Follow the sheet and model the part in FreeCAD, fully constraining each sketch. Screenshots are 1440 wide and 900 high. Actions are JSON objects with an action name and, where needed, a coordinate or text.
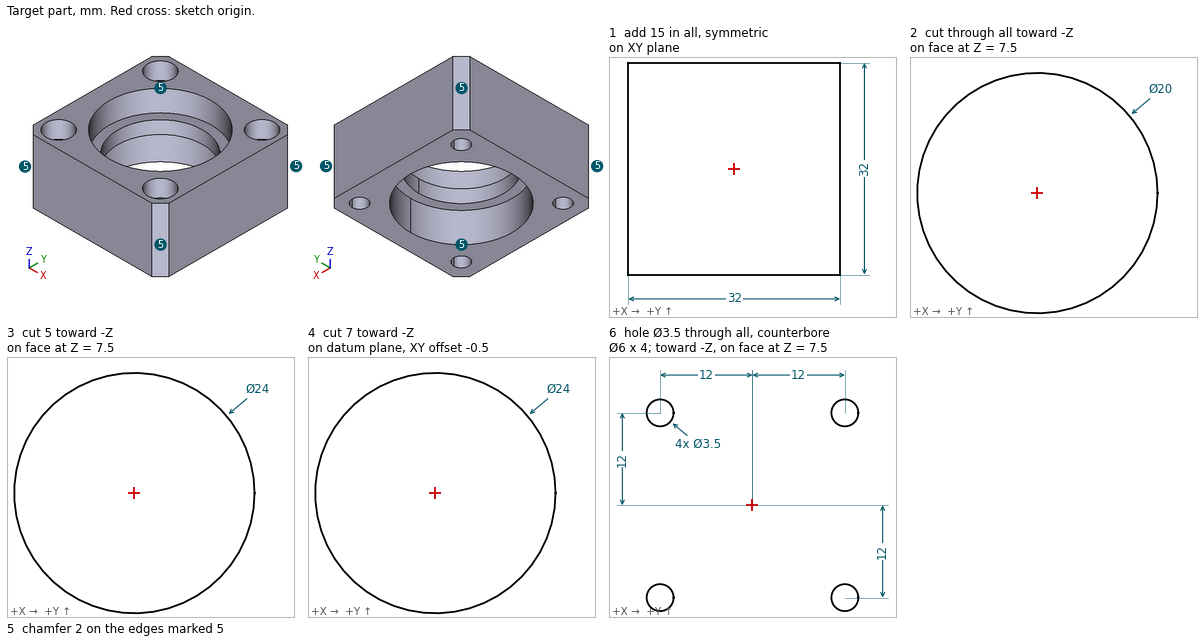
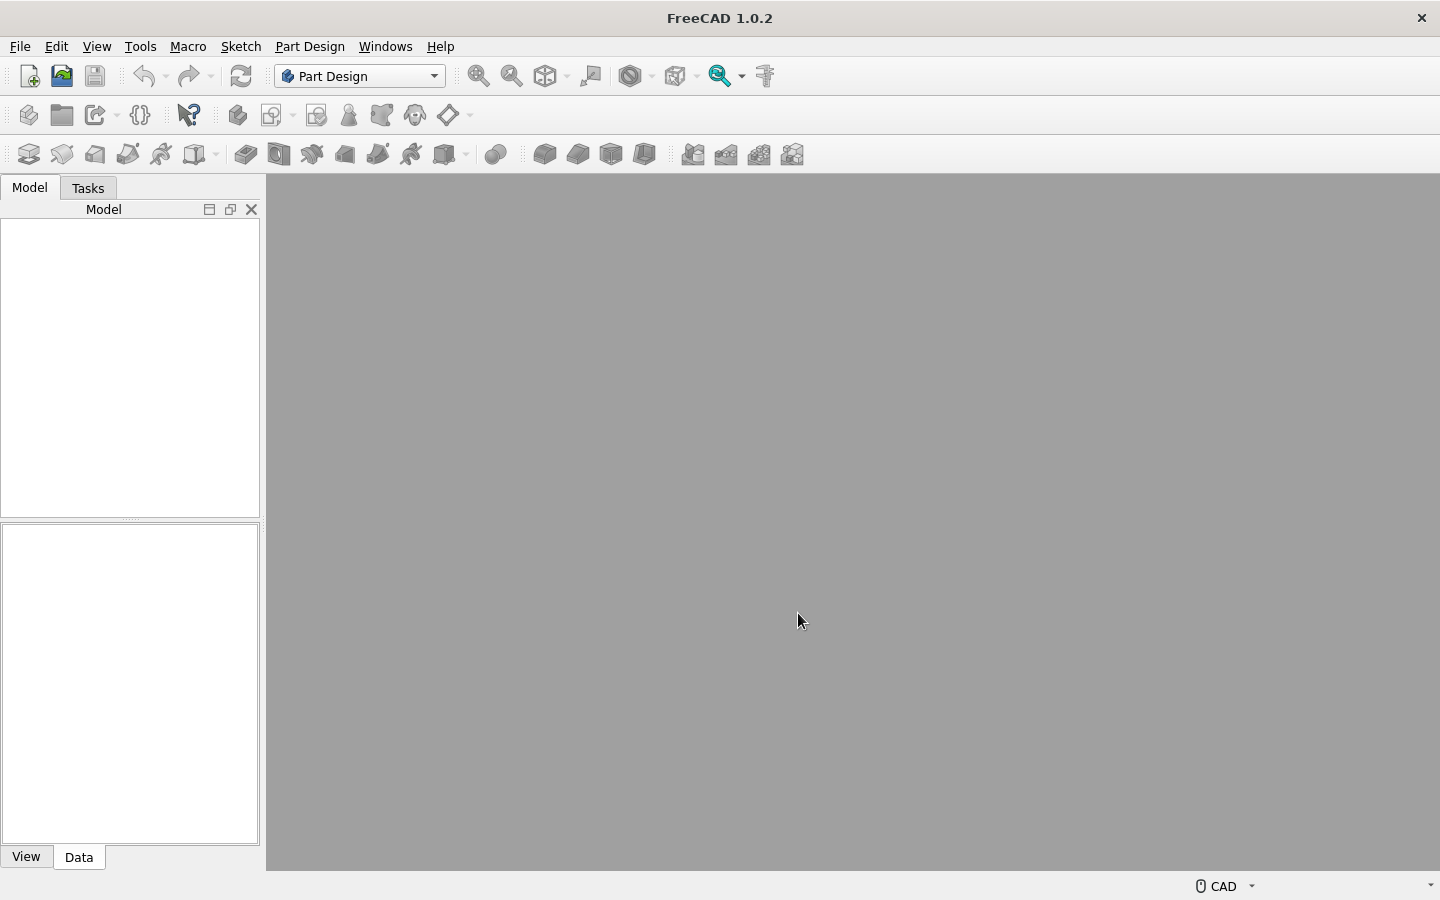
{"action": "left_click", "coordinate": [29, 76]}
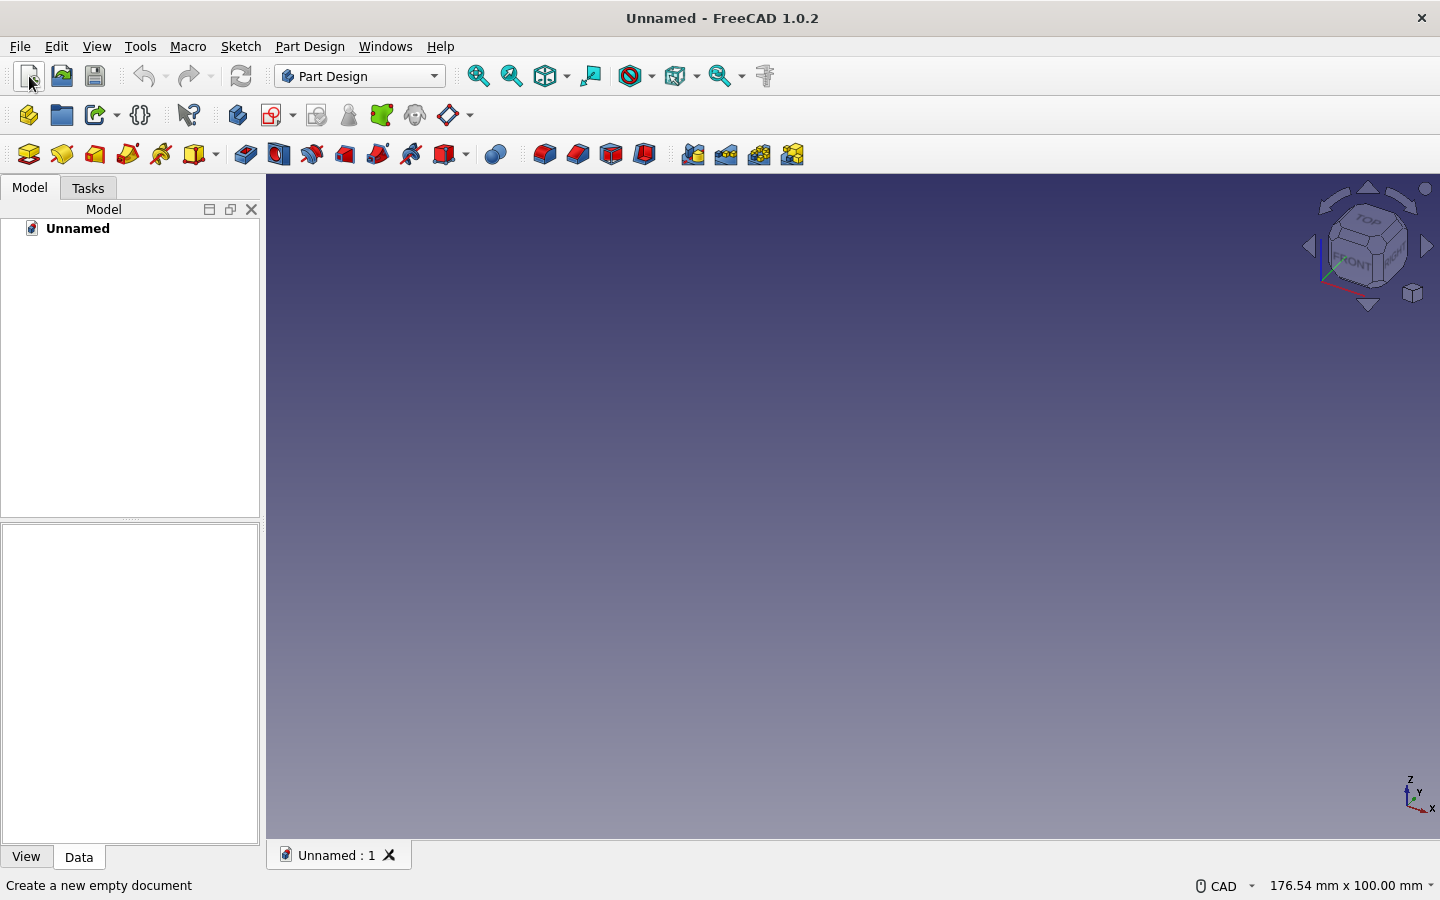
{"action": "left_click", "coordinate": [270, 116]}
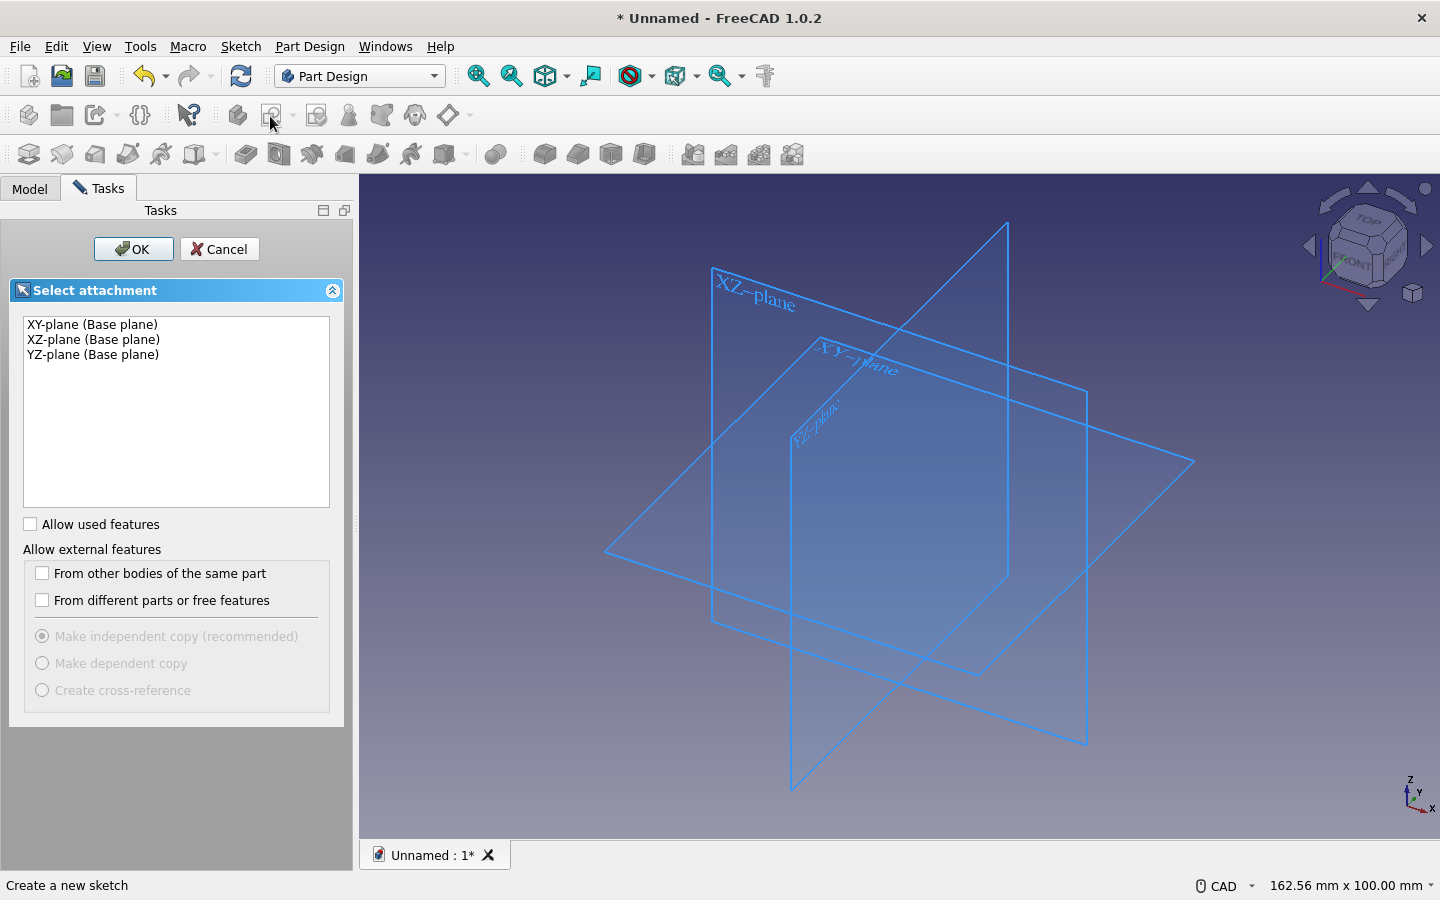
{"action": "left_click", "coordinate": [84, 324]}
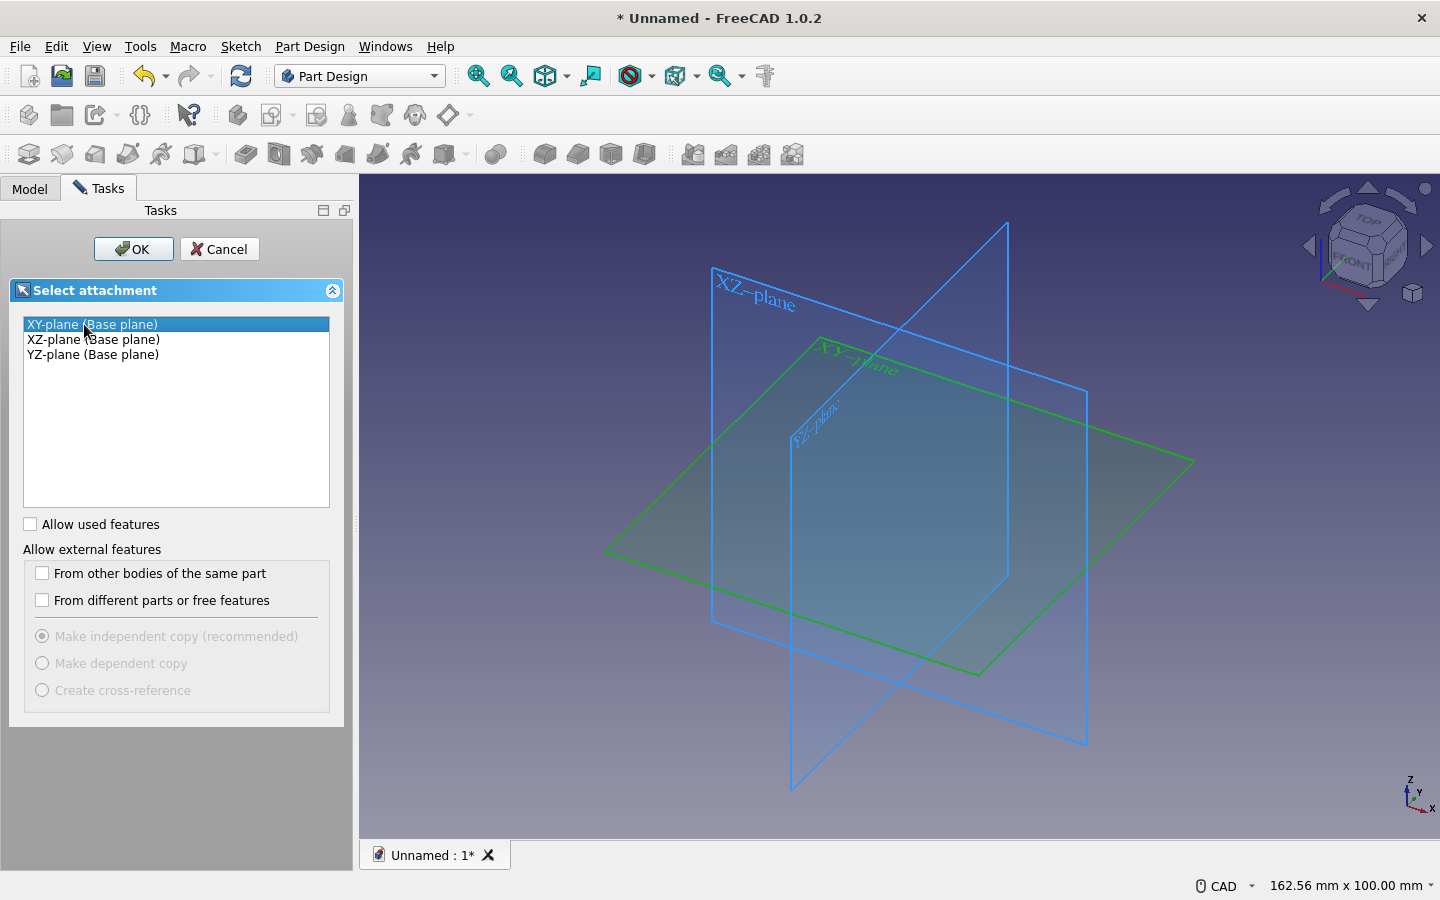
{"action": "left_click", "coordinate": [134, 249]}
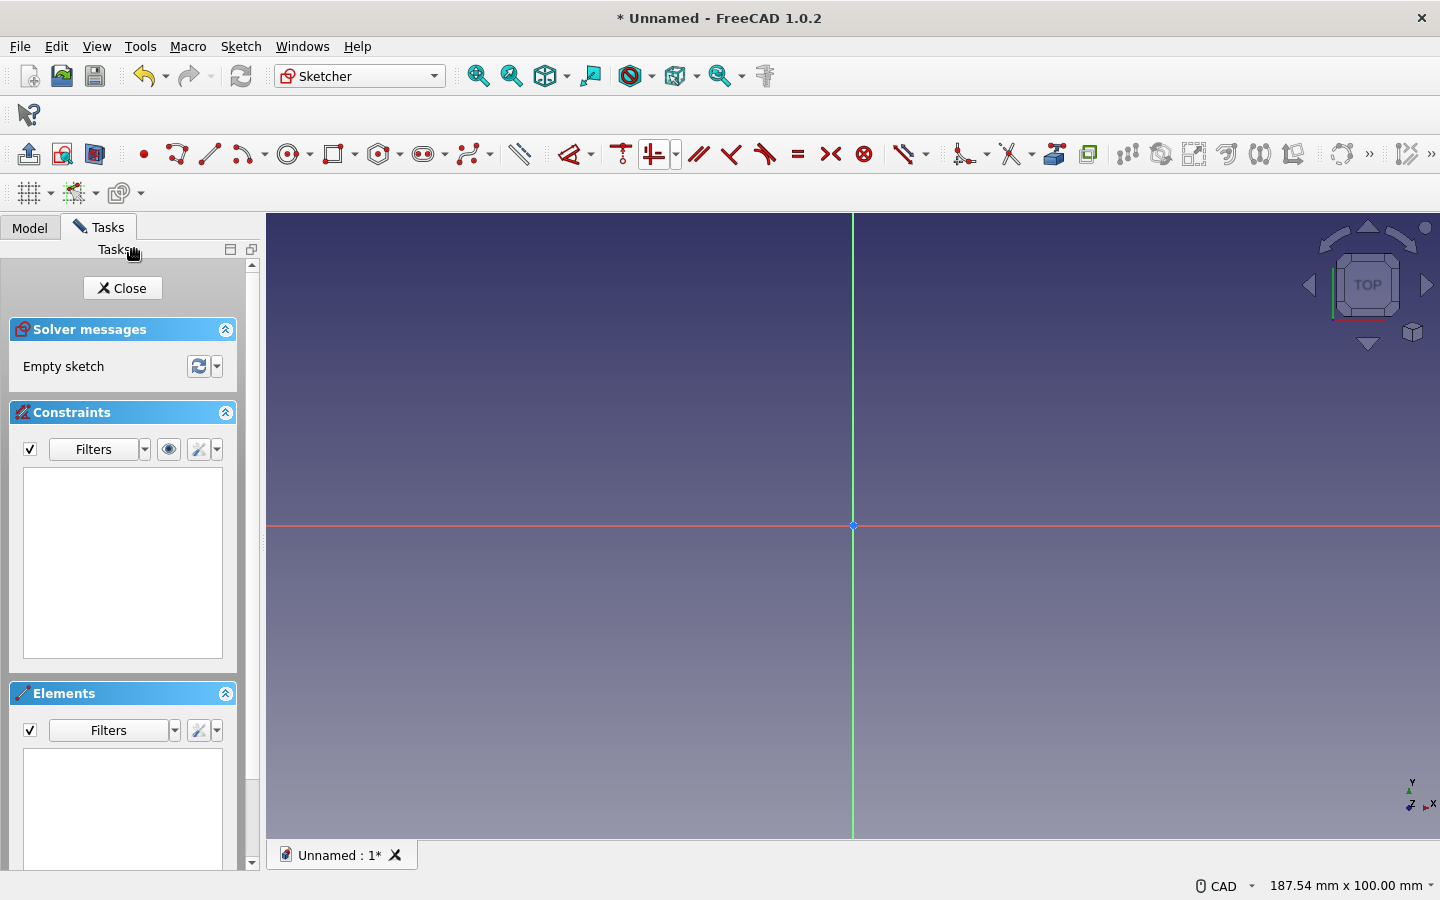
{"action": "scroll", "coordinate": [936, 526], "scroll_direction": "up", "scroll_amount": 3}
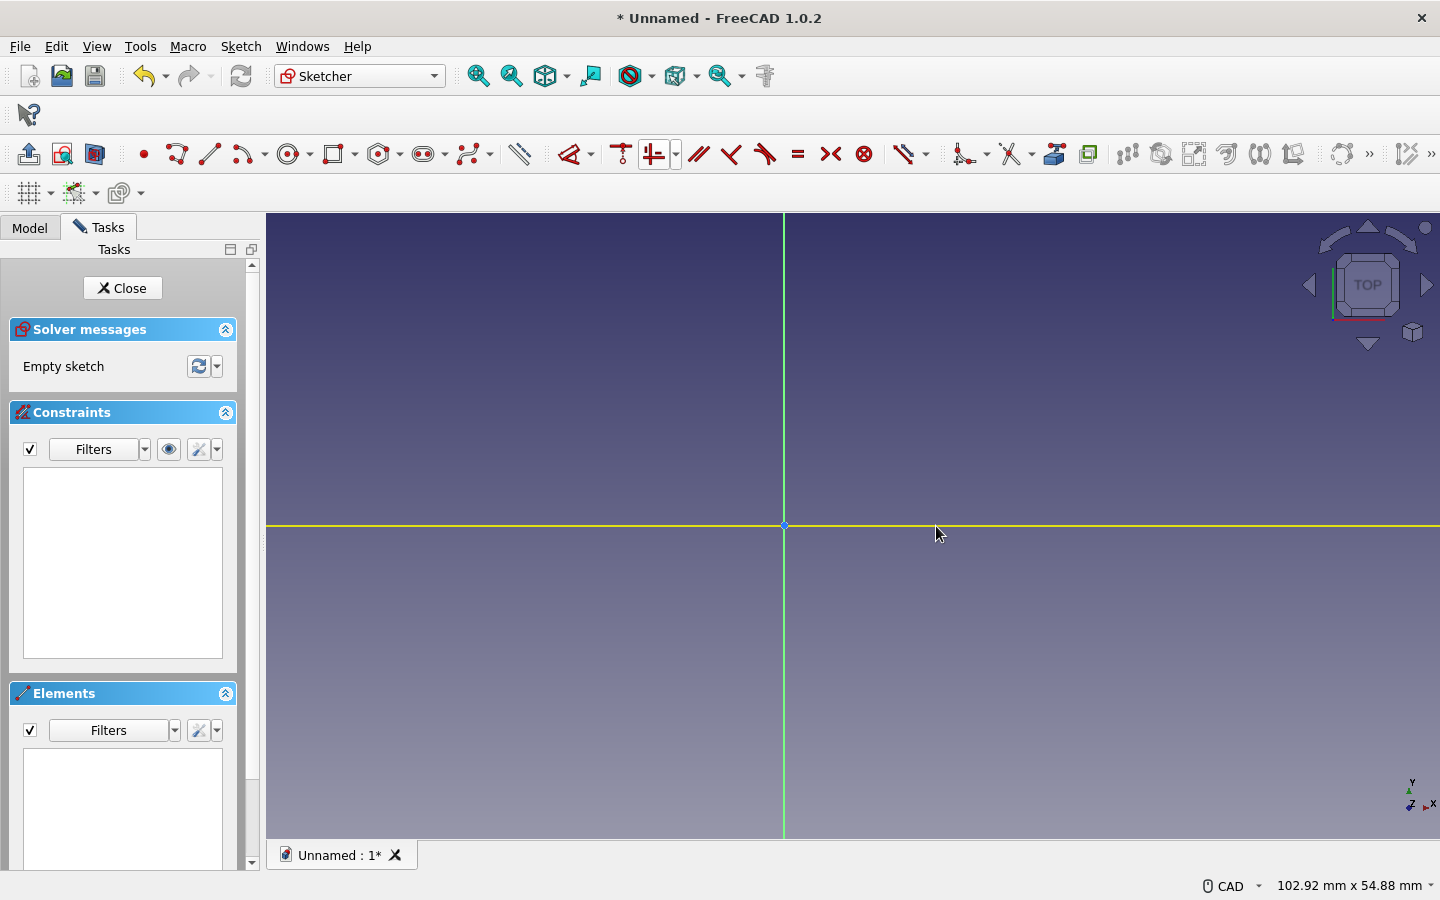
{"action": "key", "text": "g v"}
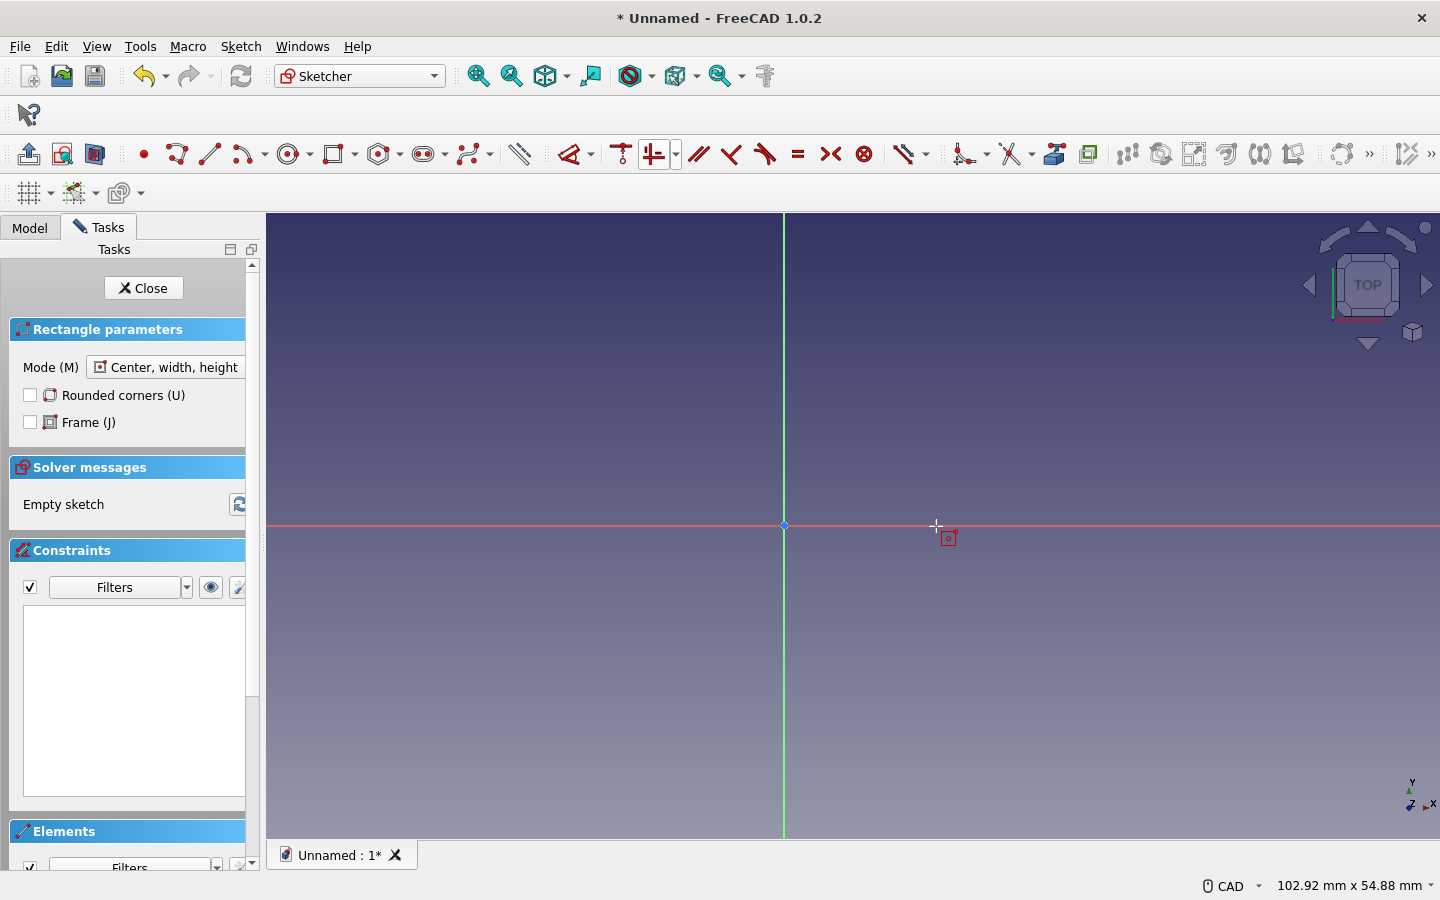
{"action": "left_click", "coordinate": [784, 526]}
{"action": "left_click", "coordinate": [967, 343]}
{"action": "key", "text": "Escape"}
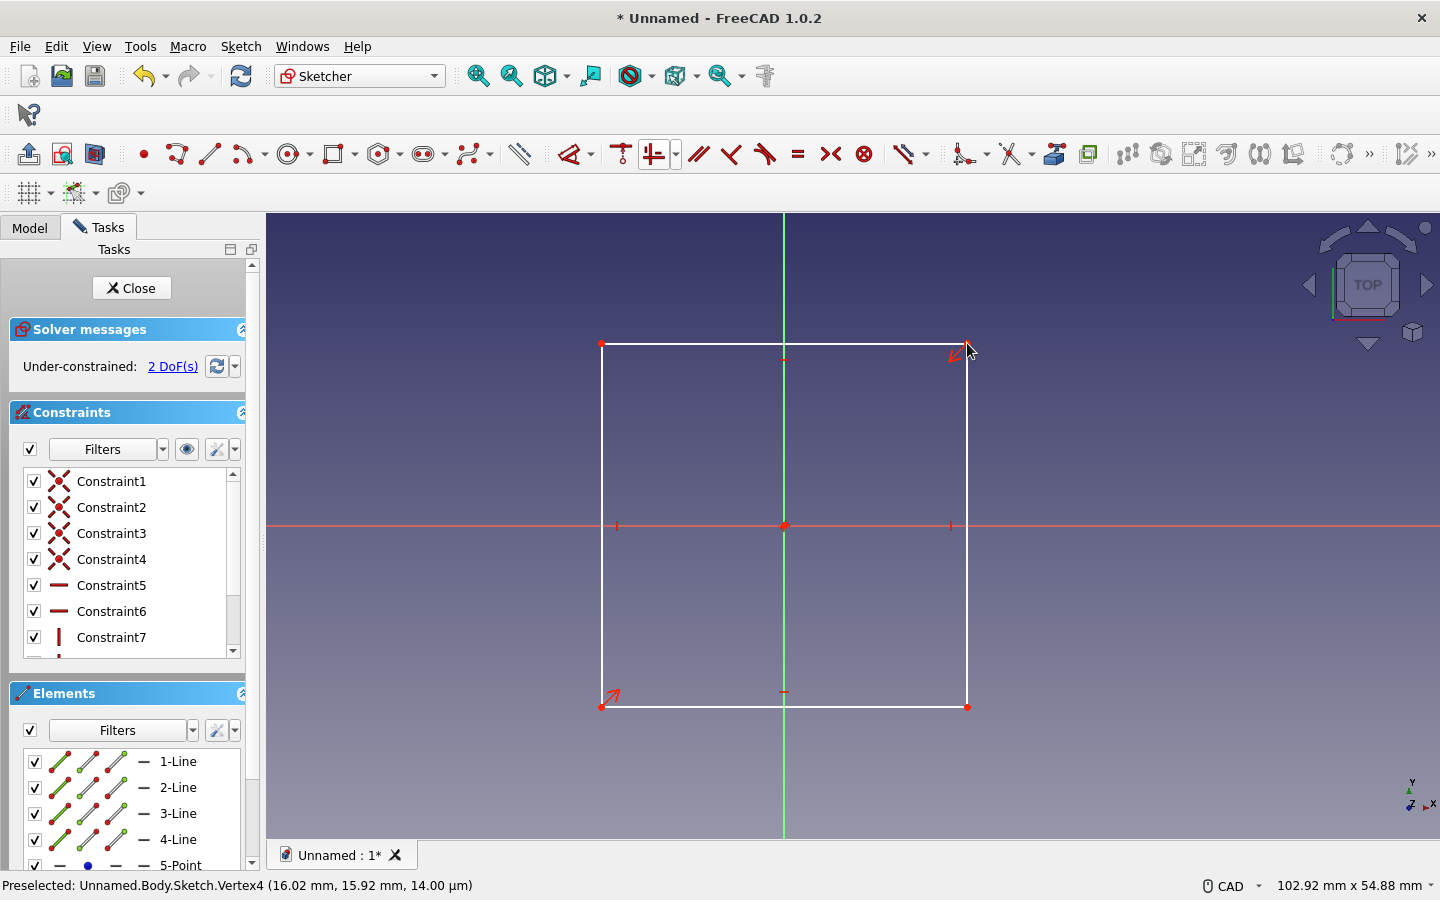
{"action": "left_click", "coordinate": [711, 707]}